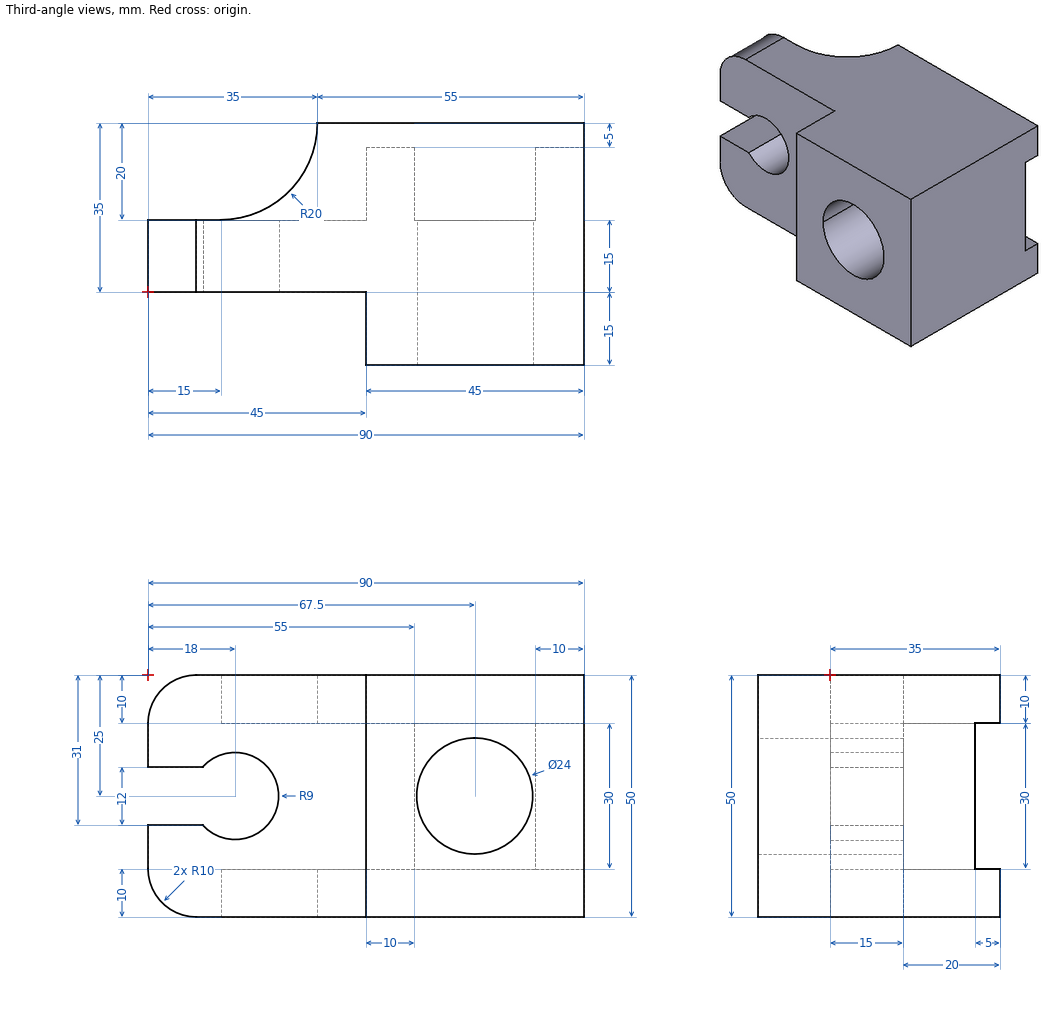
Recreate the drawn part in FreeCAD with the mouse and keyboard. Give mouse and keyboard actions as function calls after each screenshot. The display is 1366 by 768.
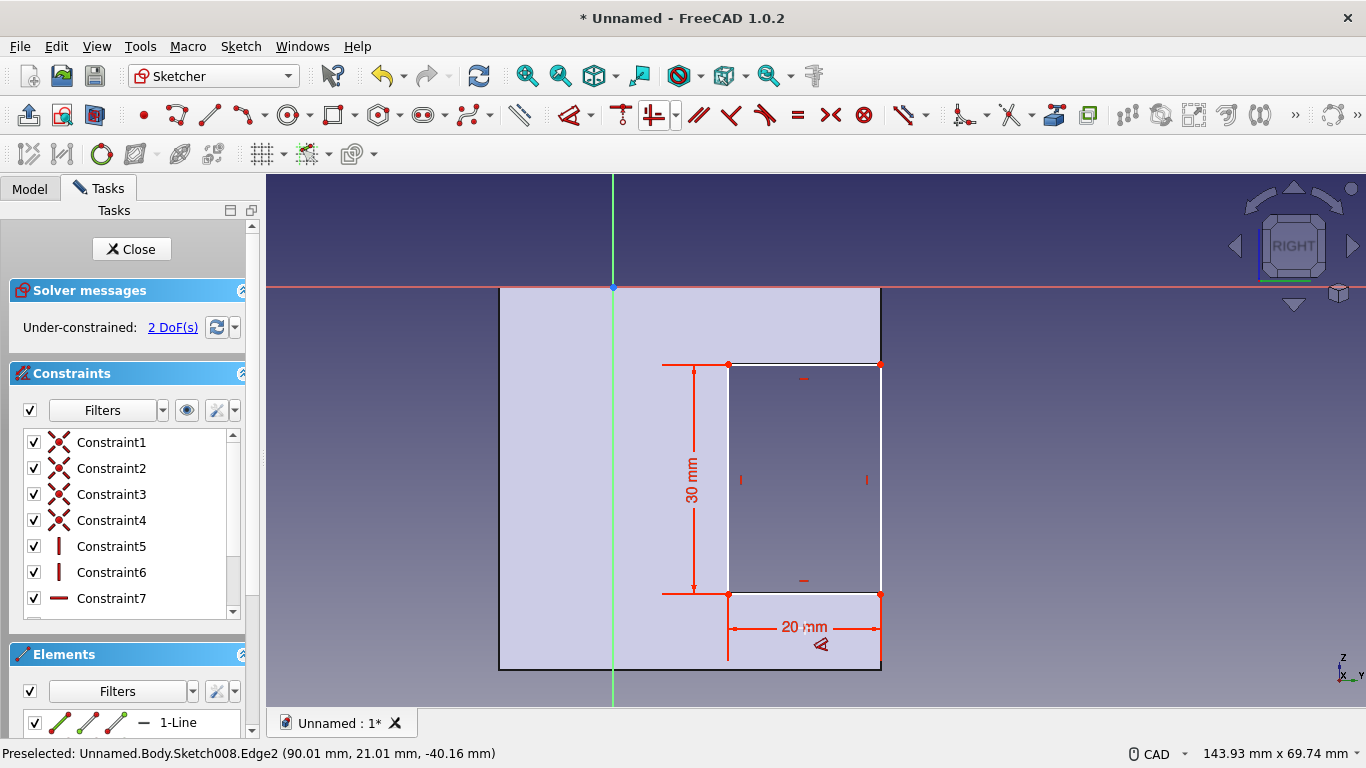
click(728, 365)
click(671, 253)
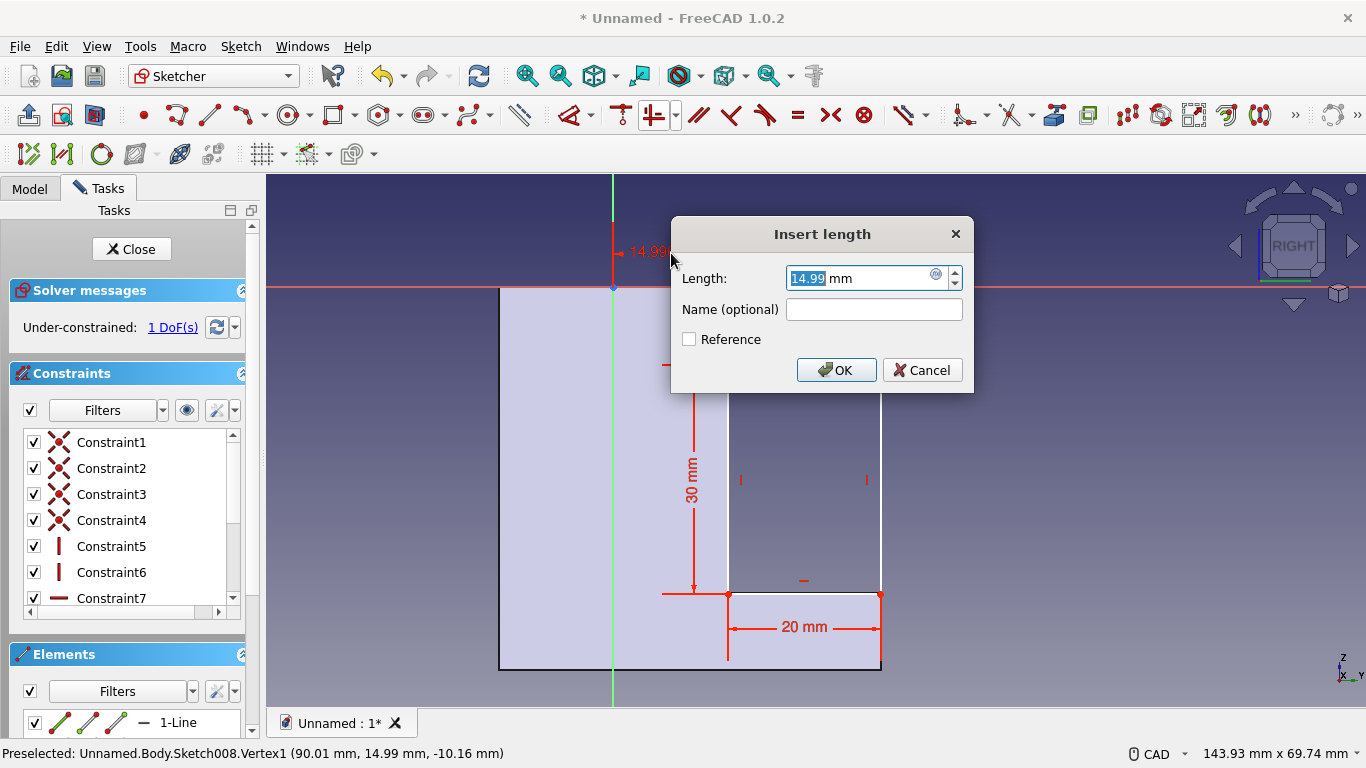
text(15)
key(Return)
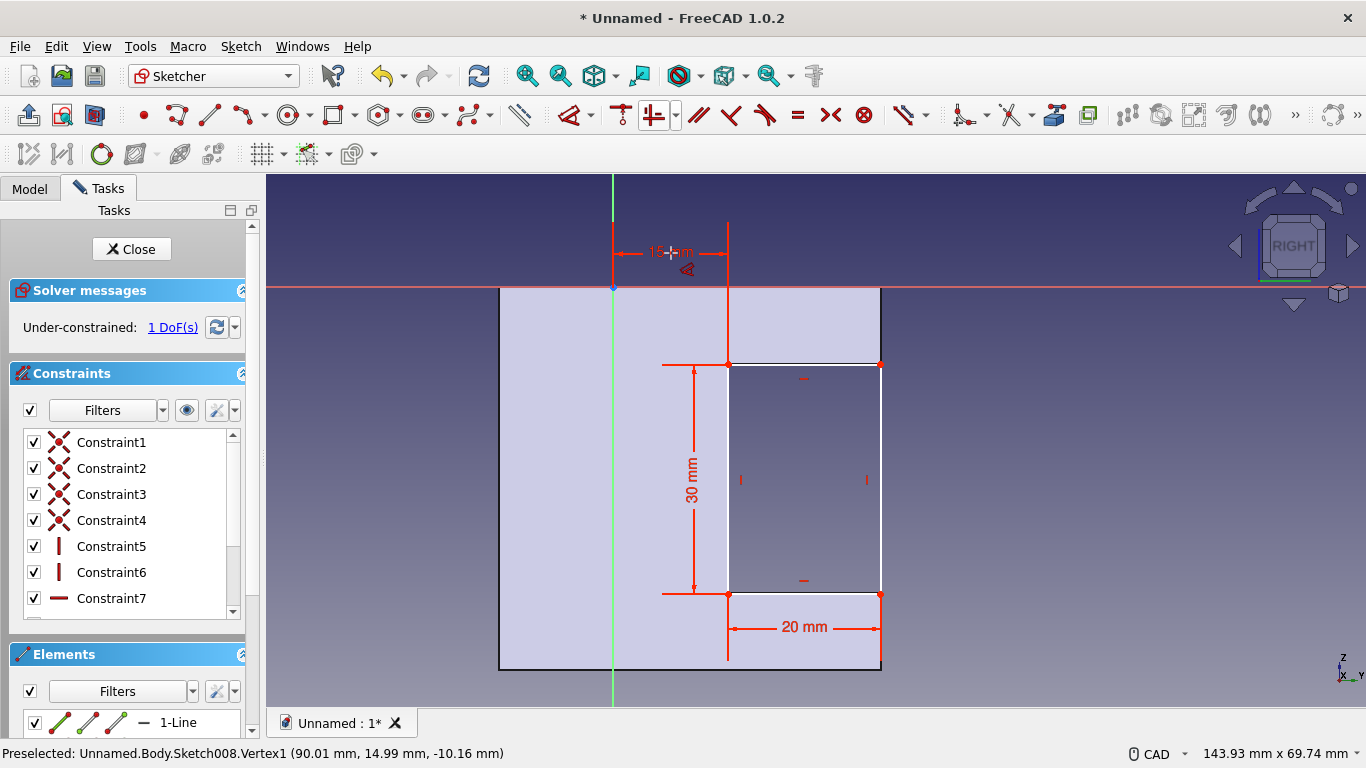
click(728, 365)
click(579, 326)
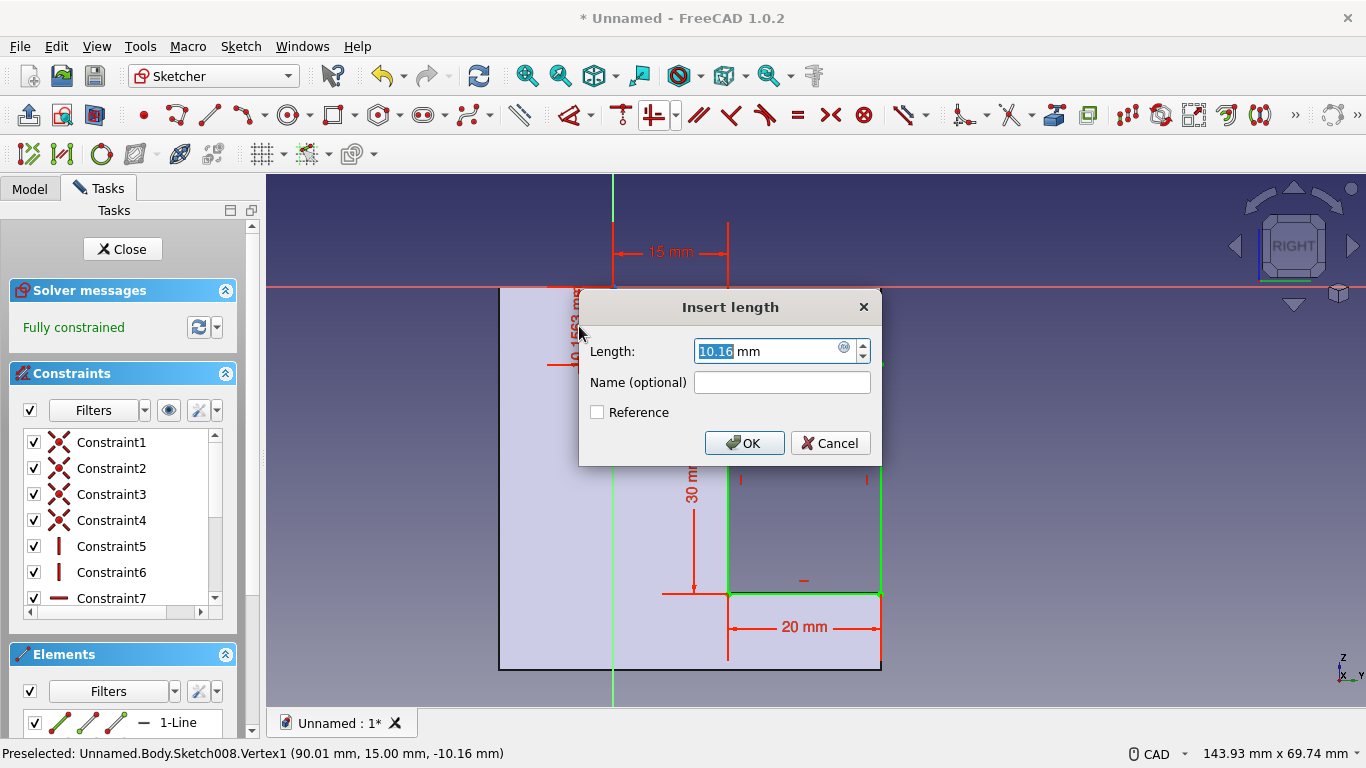
text(10)
key(Return)
key(Escape)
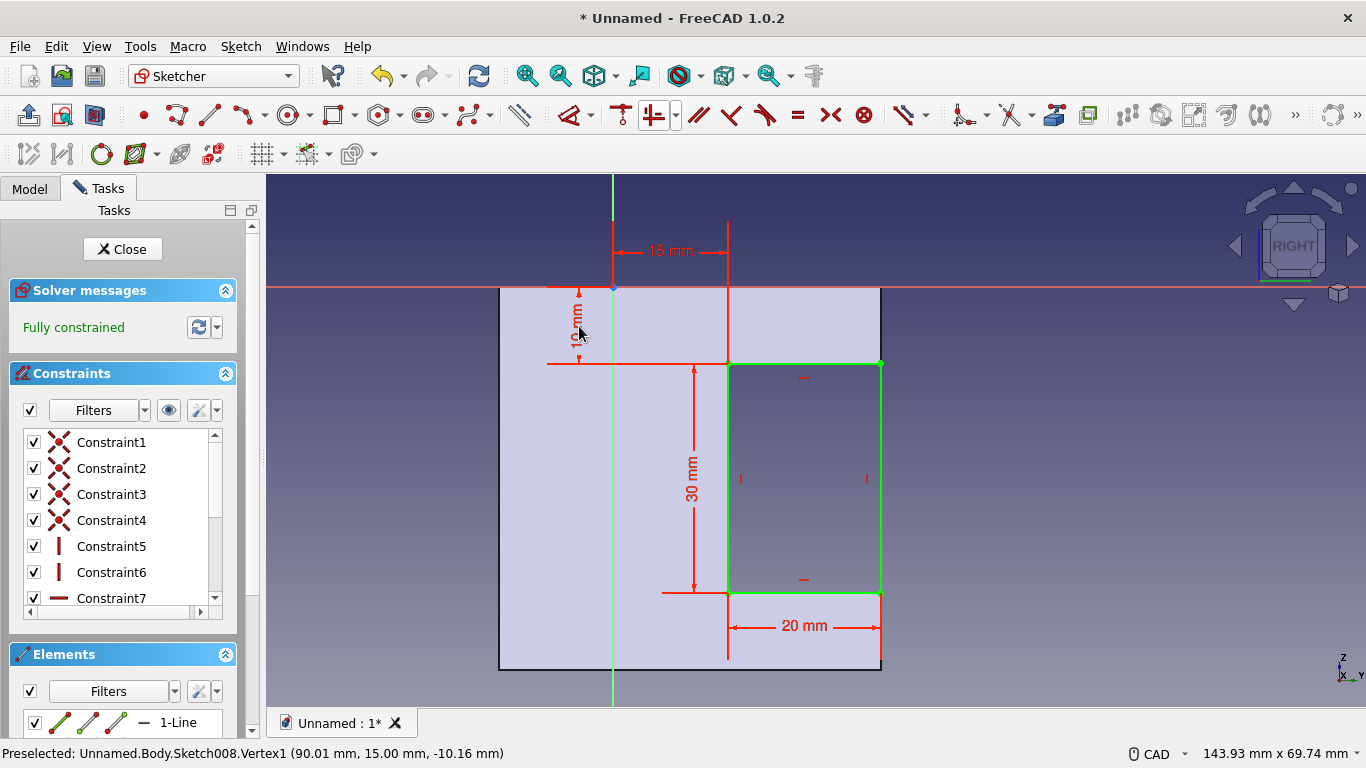
click(123, 249)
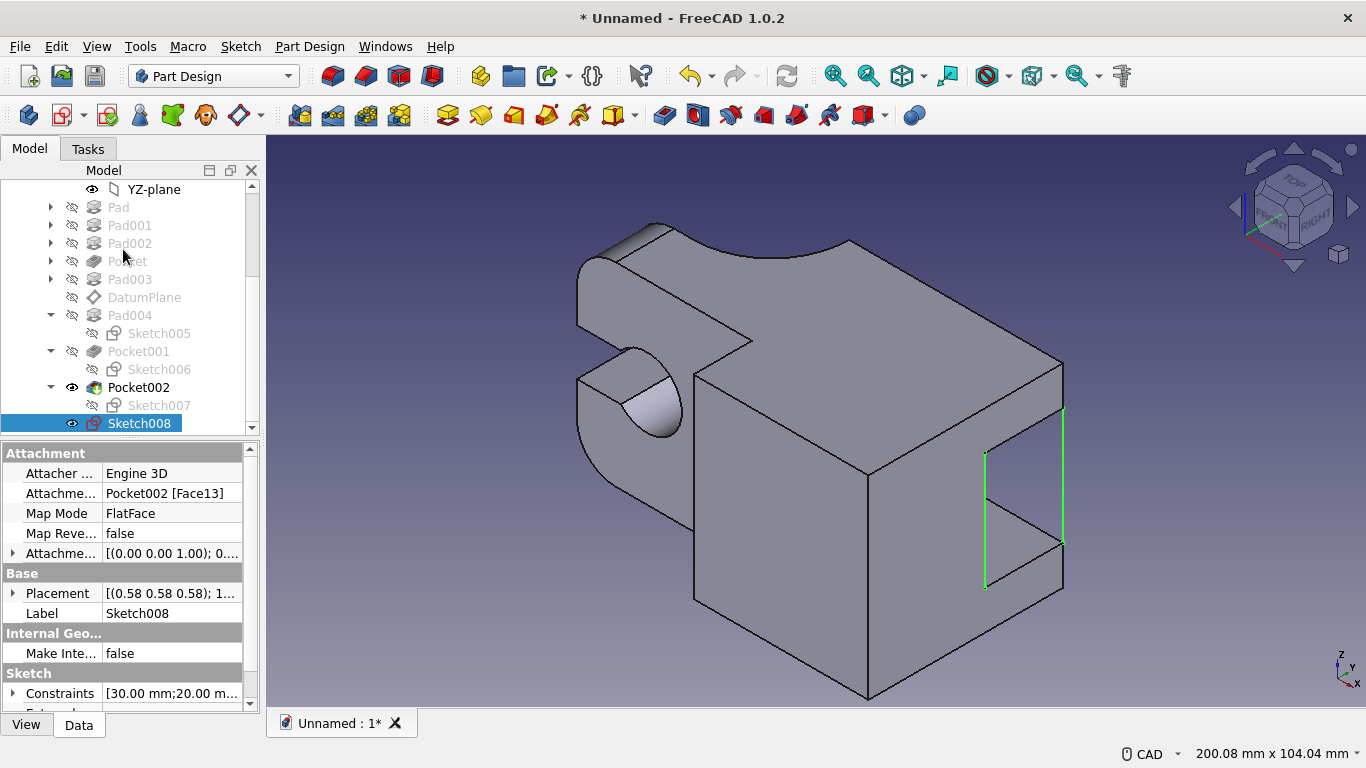
click(448, 116)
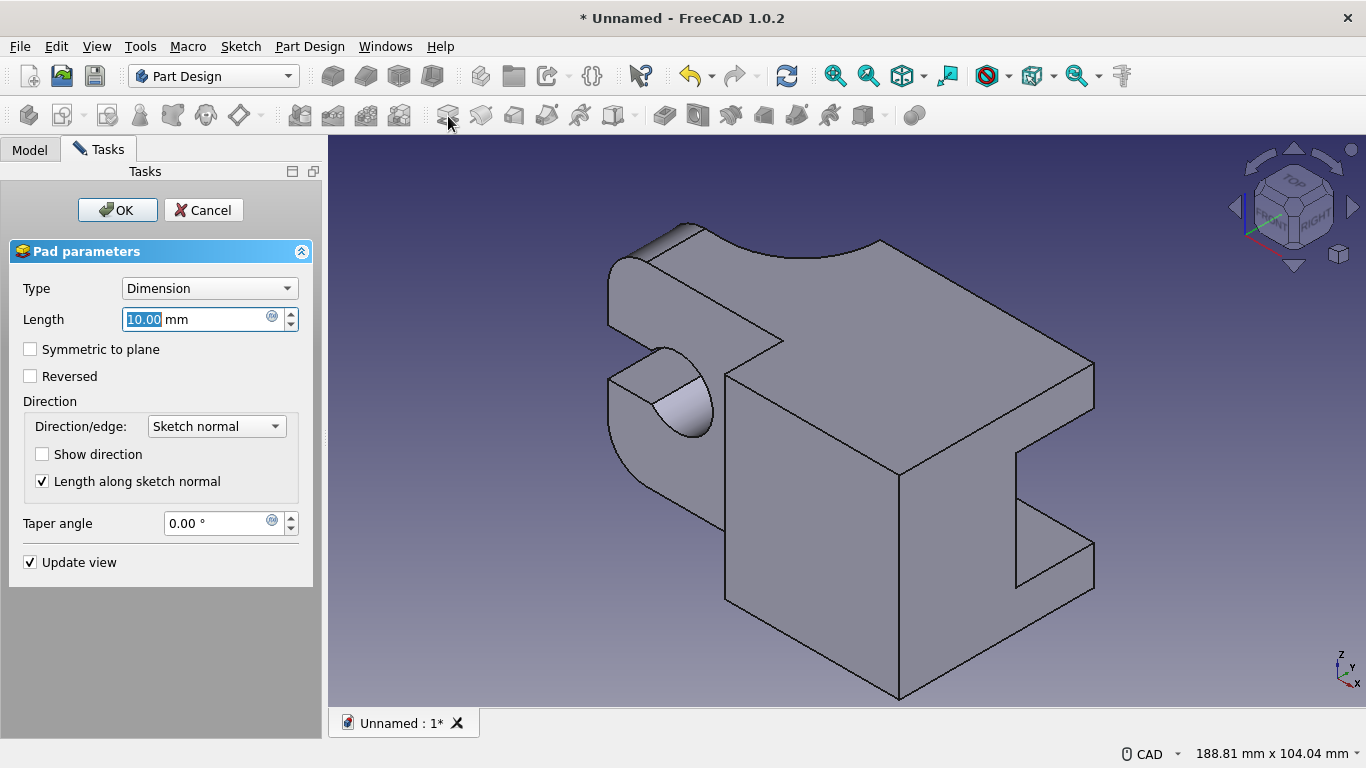
text(10)
key(Tab)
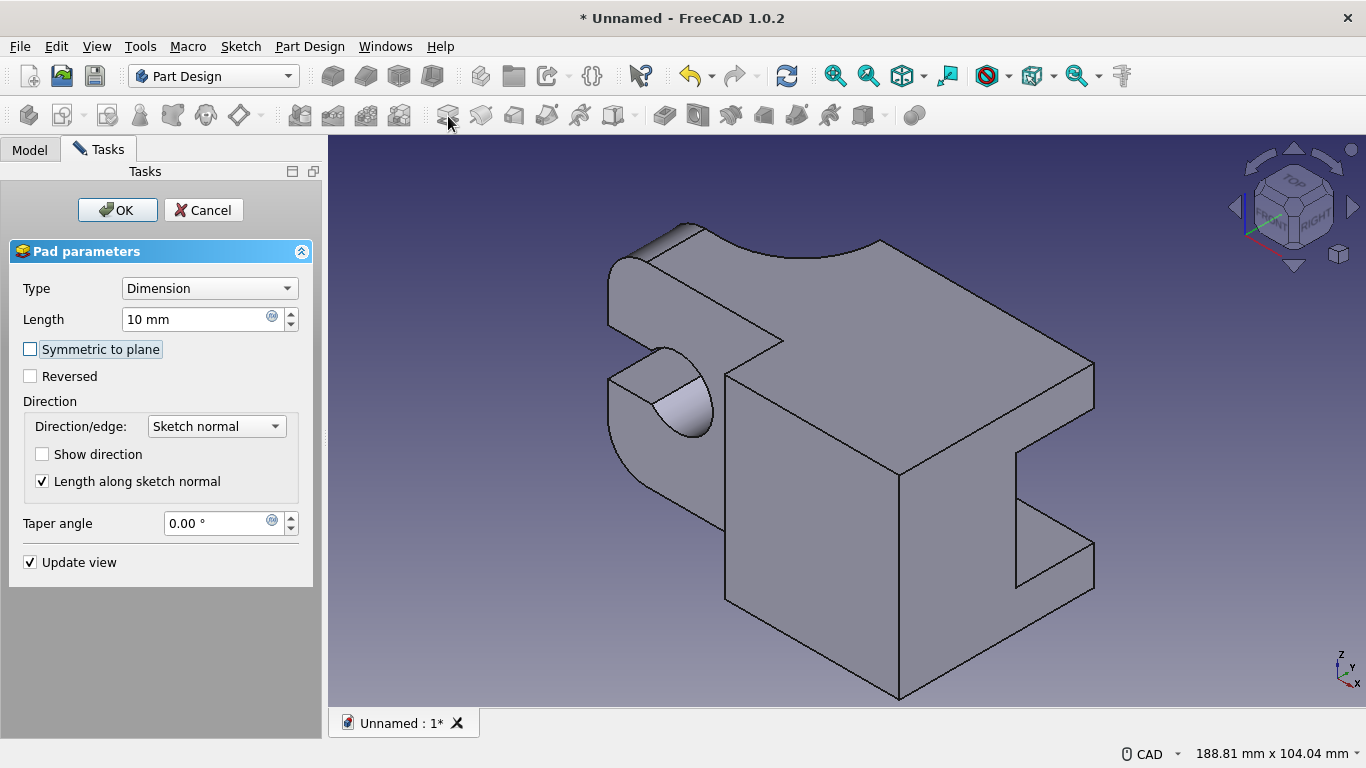
click(31, 376)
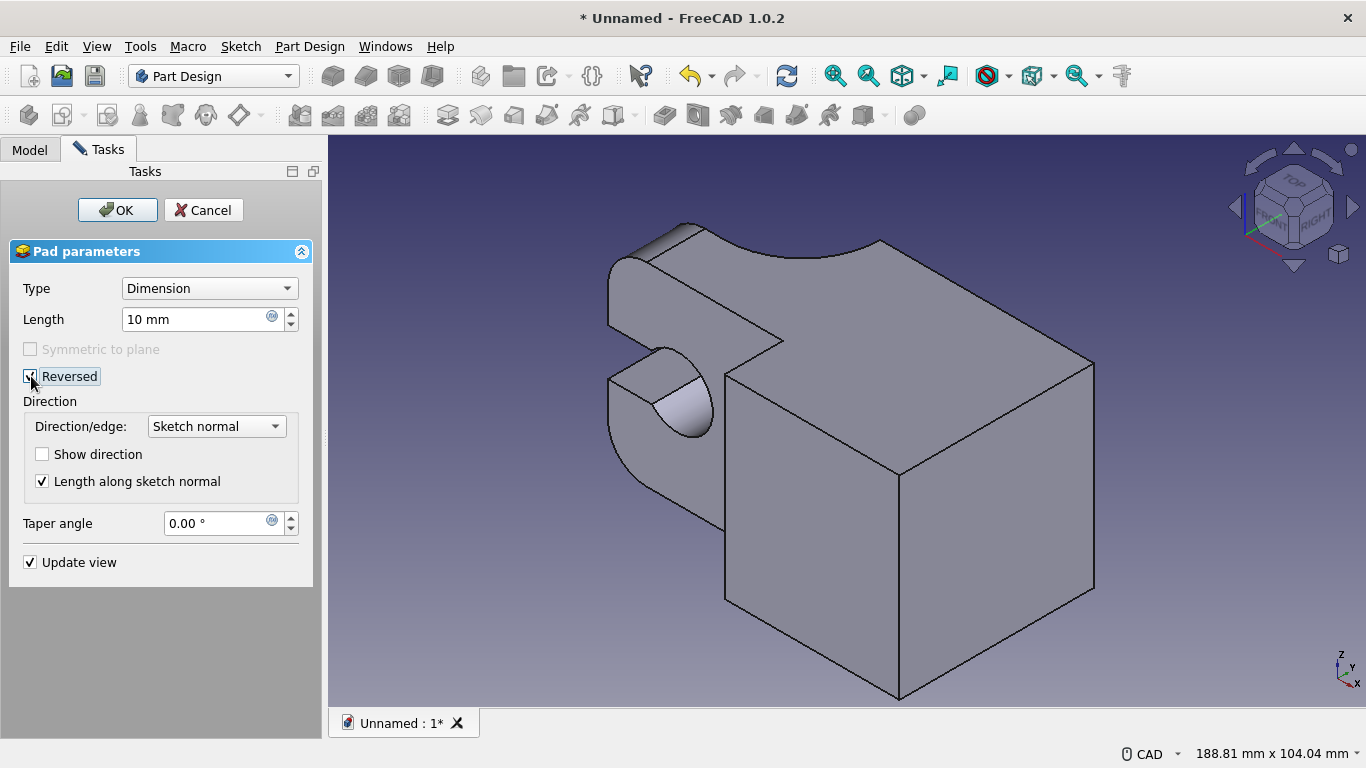
click(118, 210)